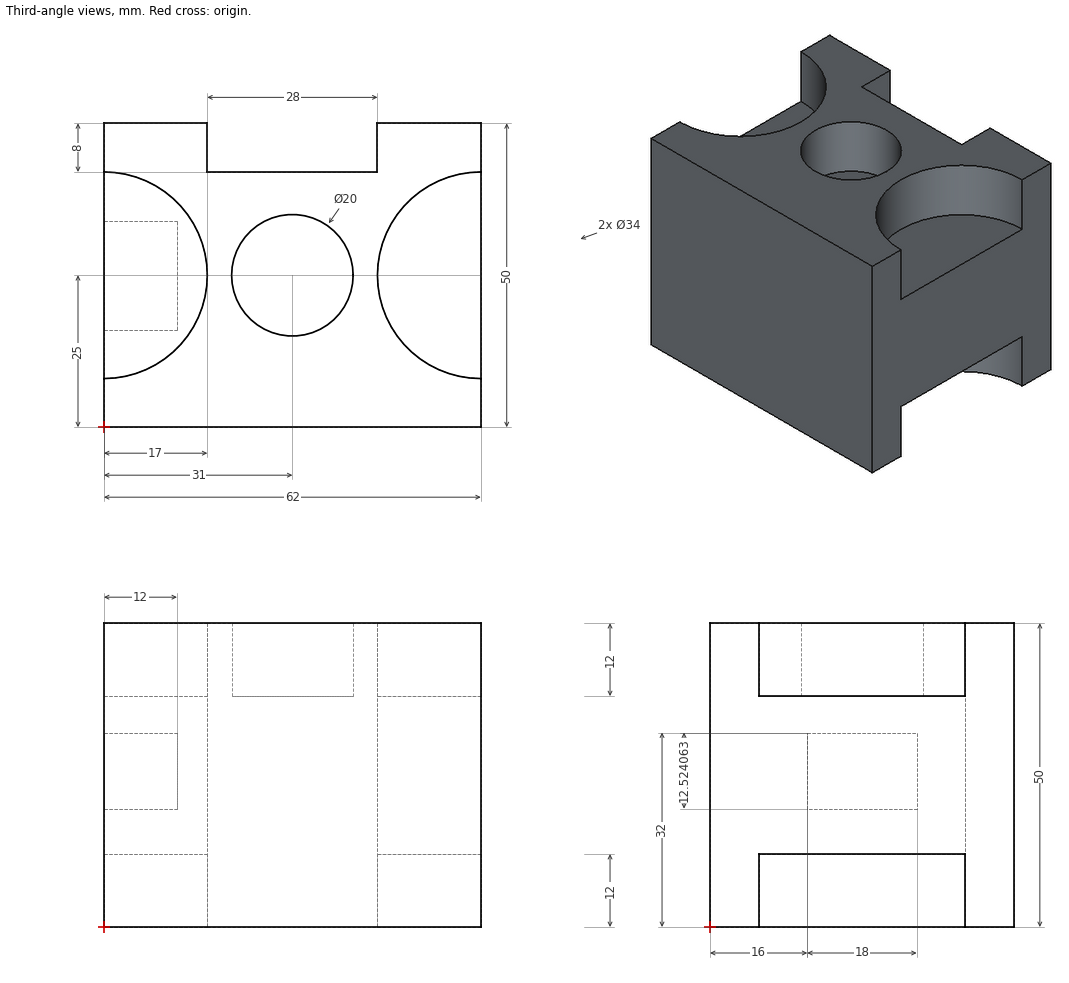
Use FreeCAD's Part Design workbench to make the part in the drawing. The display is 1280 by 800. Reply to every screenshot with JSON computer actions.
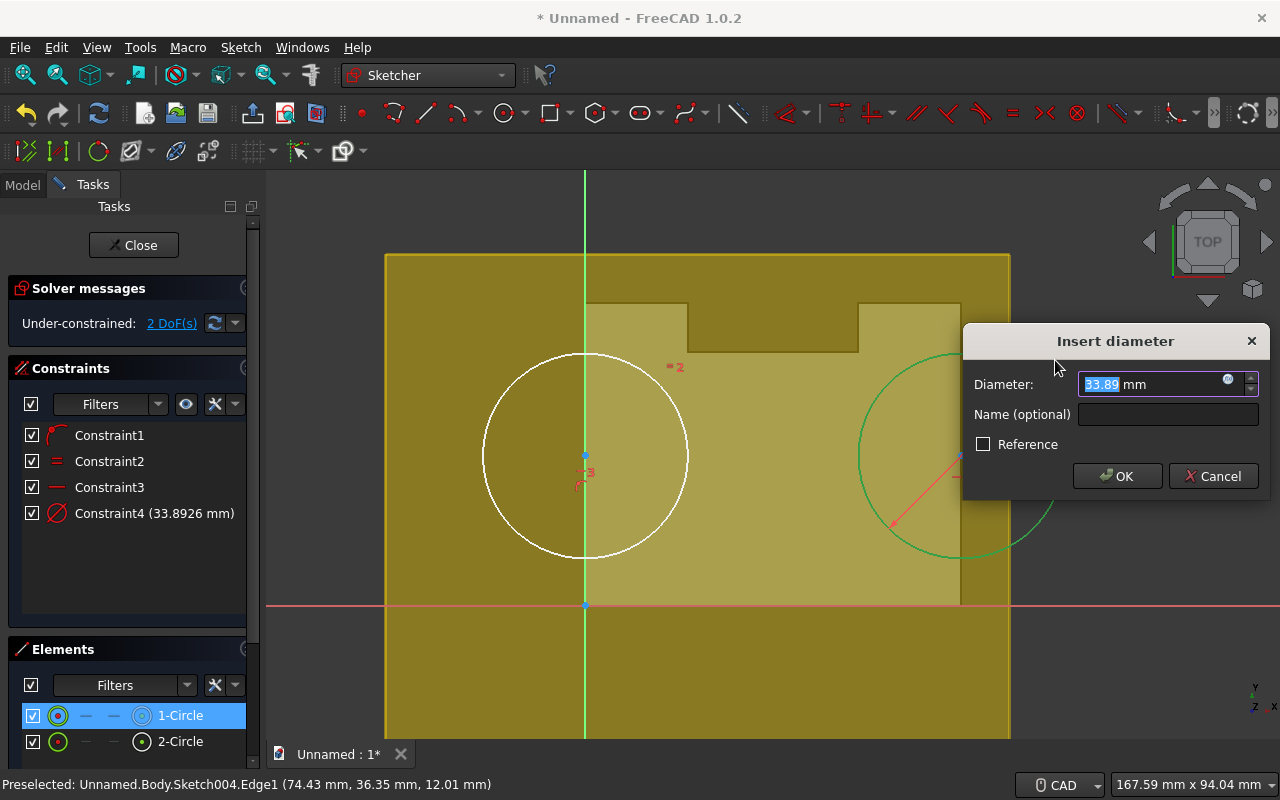
{"action": "type", "text": "34"}
{"action": "key", "text": "Return"}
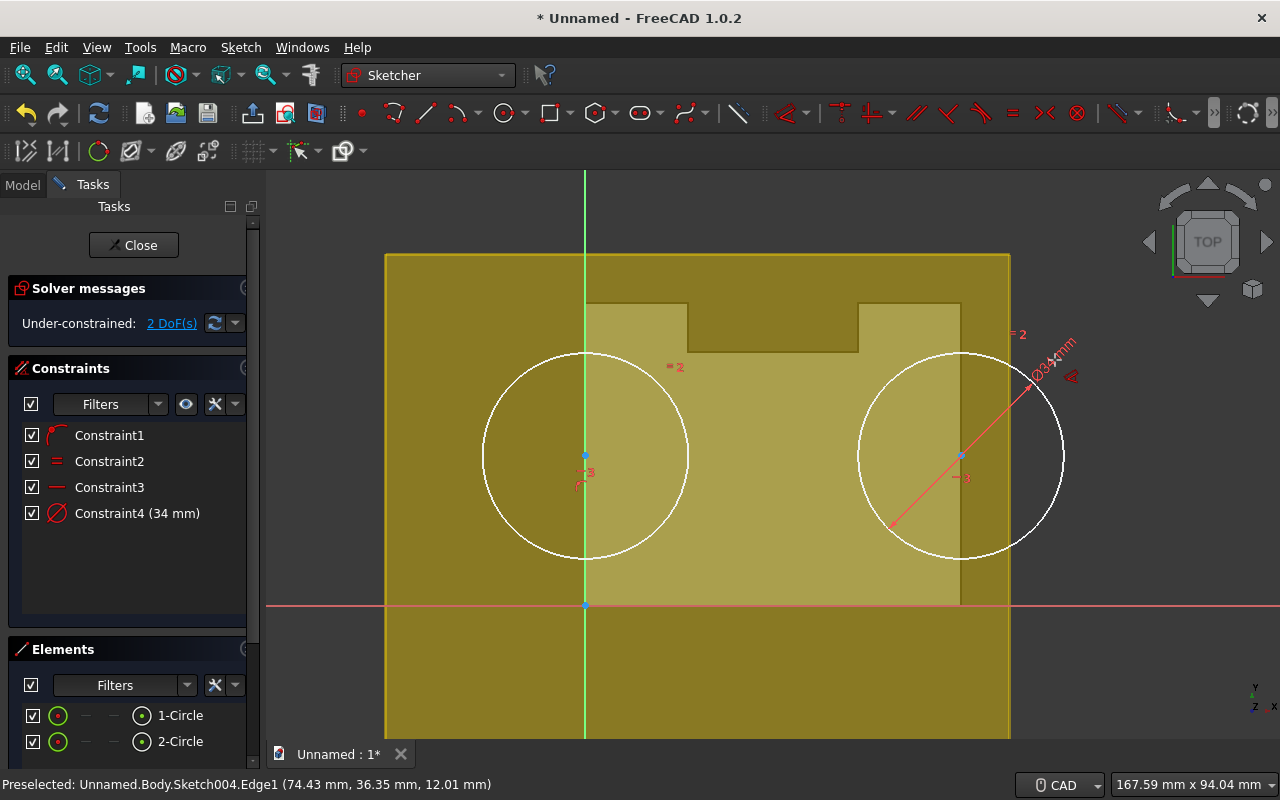
{"action": "left_click", "coordinate": [961, 456]}
{"action": "left_click", "coordinate": [773, 640]}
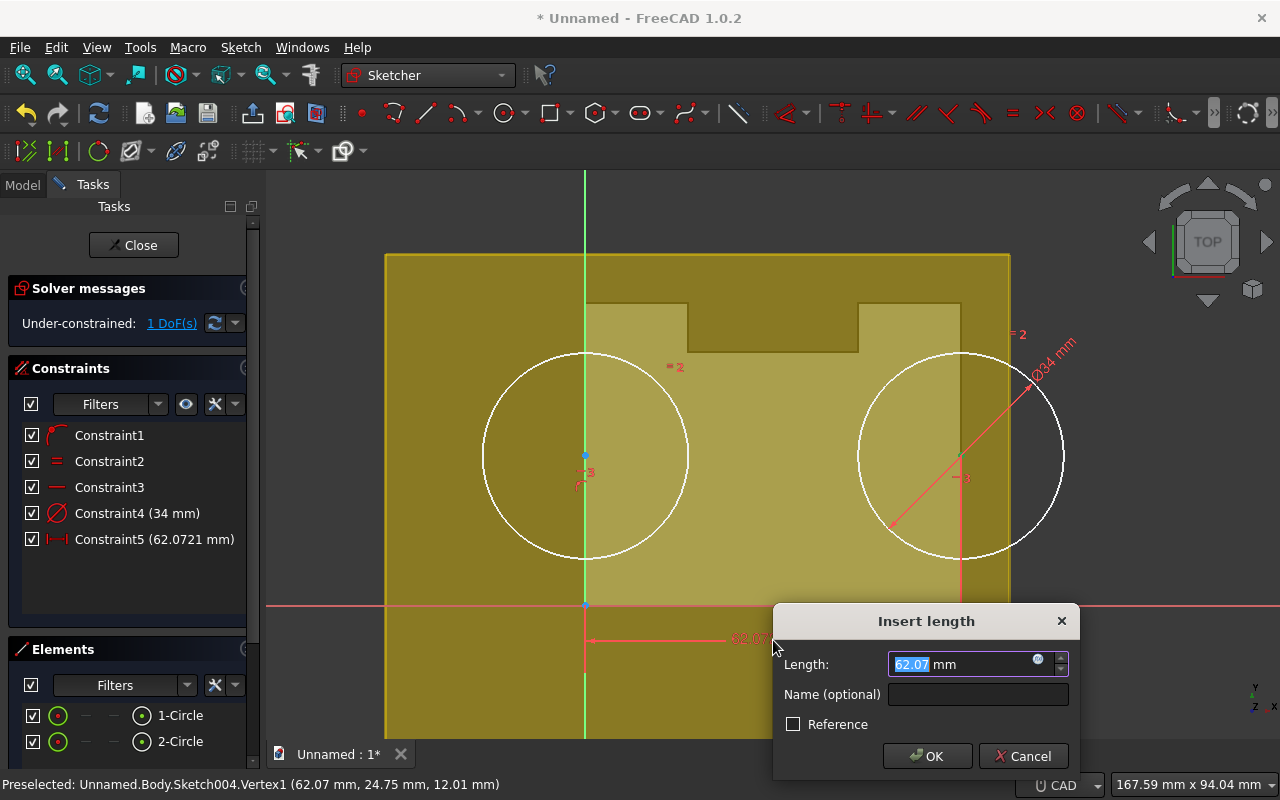
{"action": "type", "text": "62"}
{"action": "key", "text": "Return"}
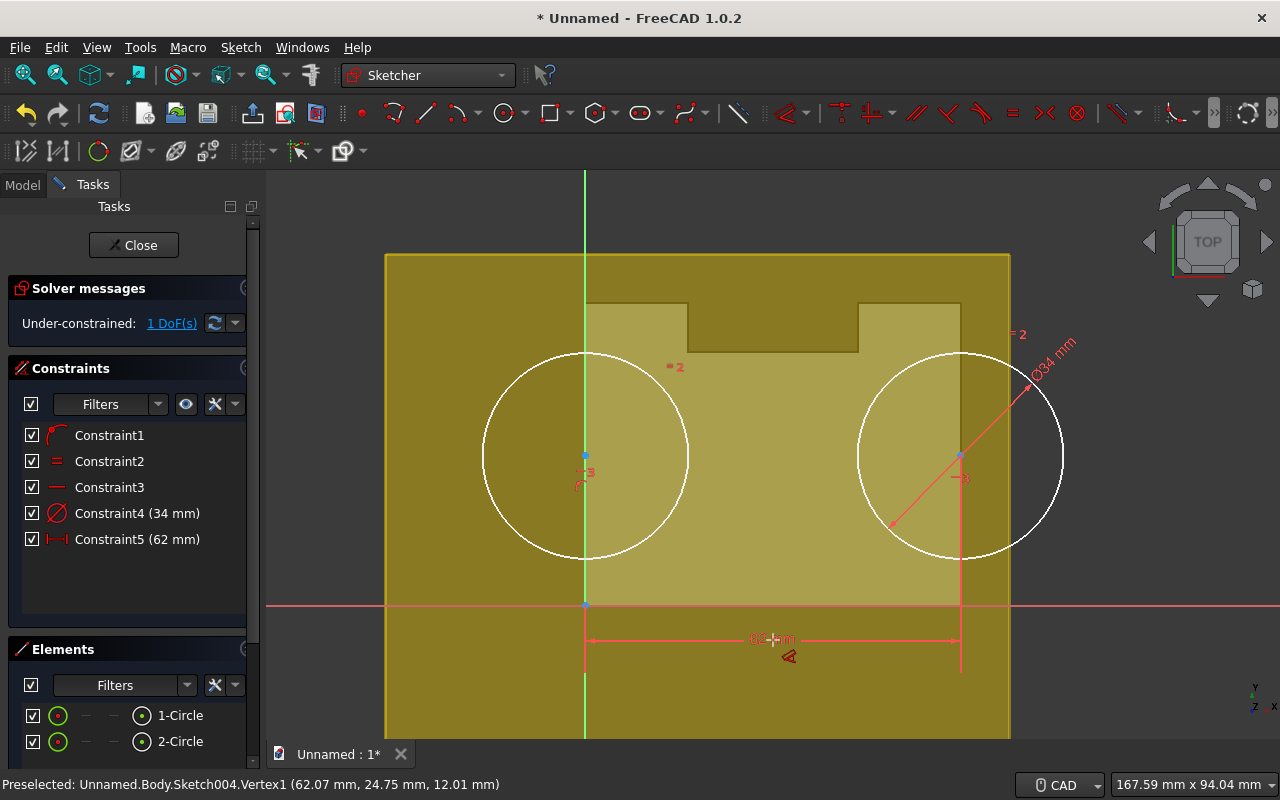
{"action": "left_click", "coordinate": [961, 456]}
{"action": "left_click", "coordinate": [995, 531]}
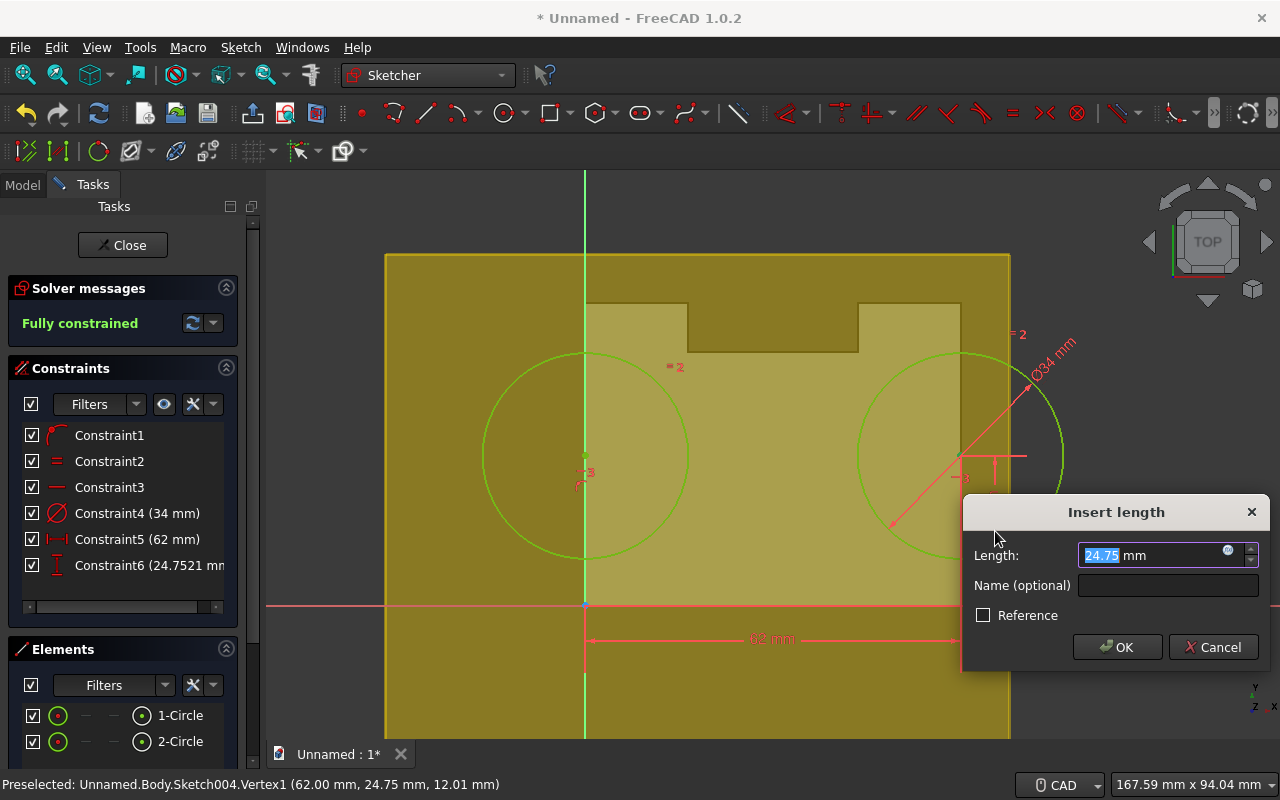
{"action": "type", "text": "25"}
{"action": "key", "text": "Return"}
{"action": "key", "text": "Escape"}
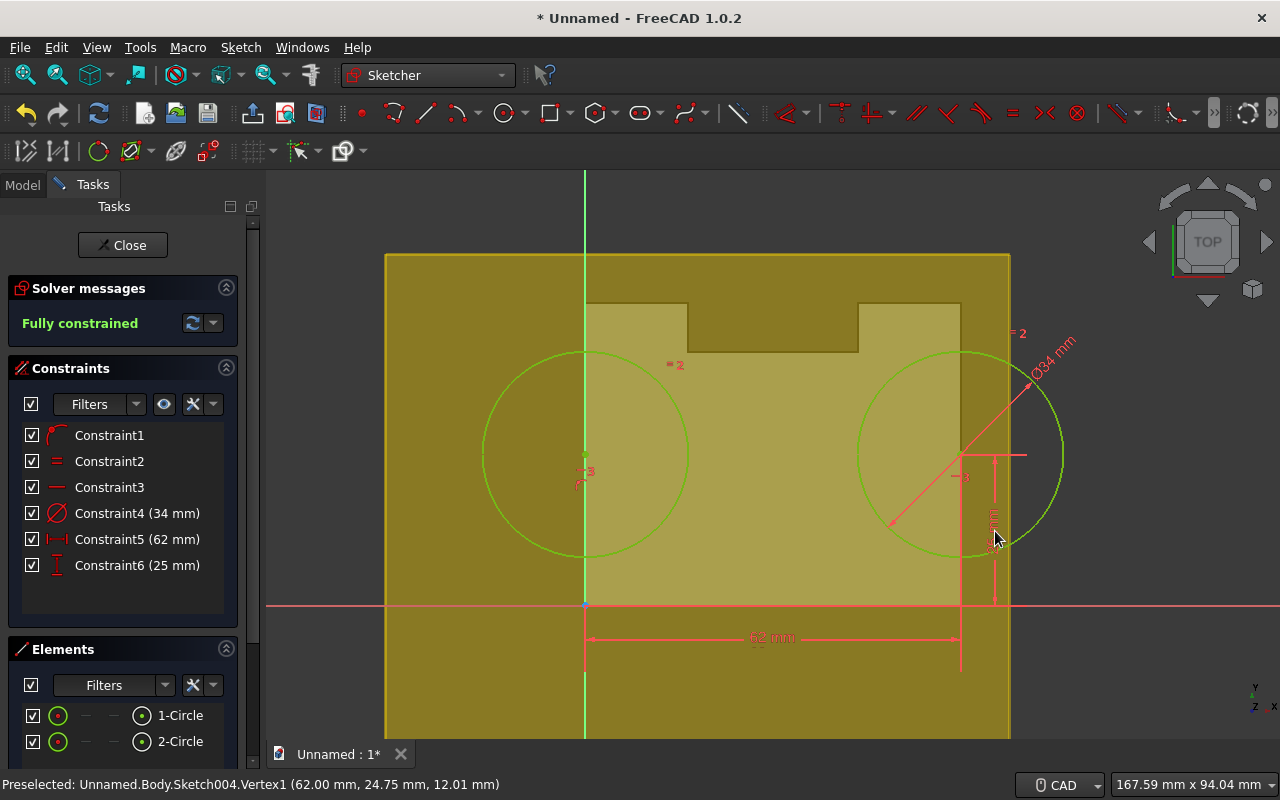
{"action": "left_click", "coordinate": [123, 245]}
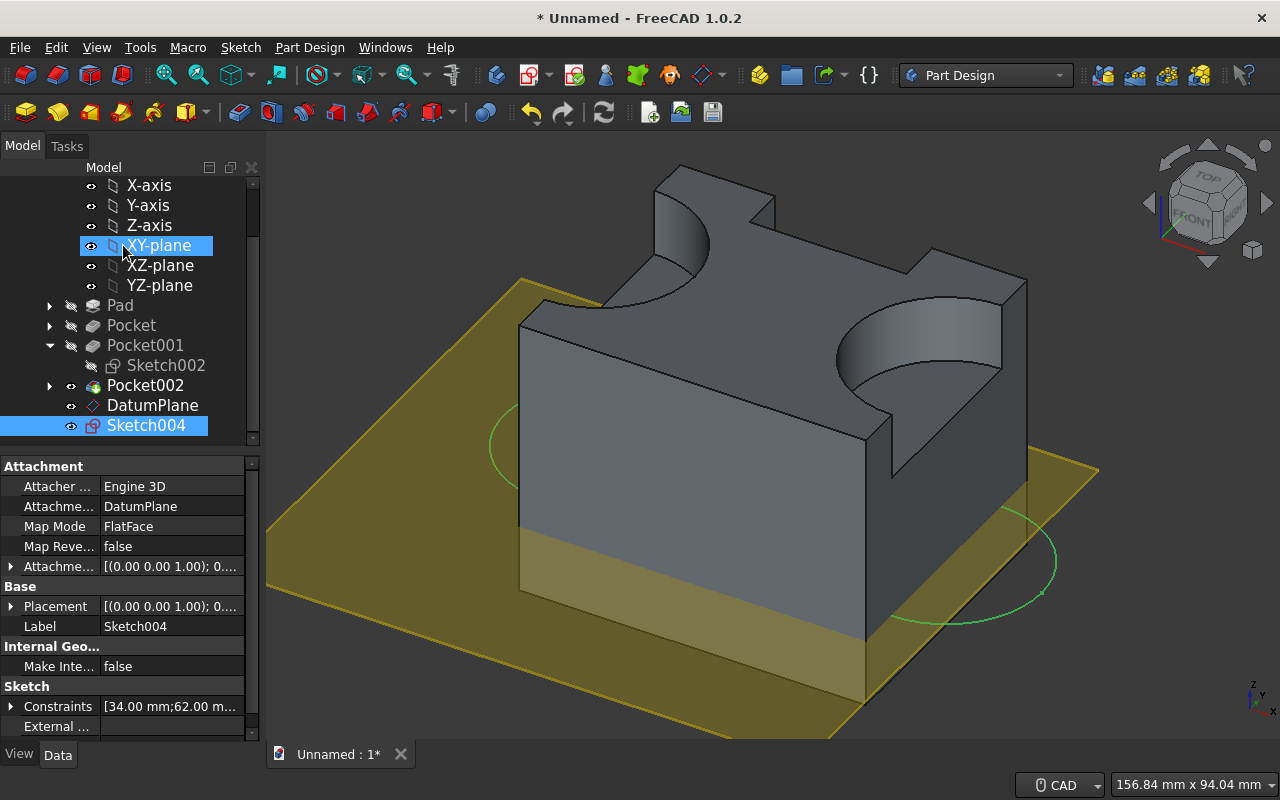
{"action": "left_click", "coordinate": [240, 112]}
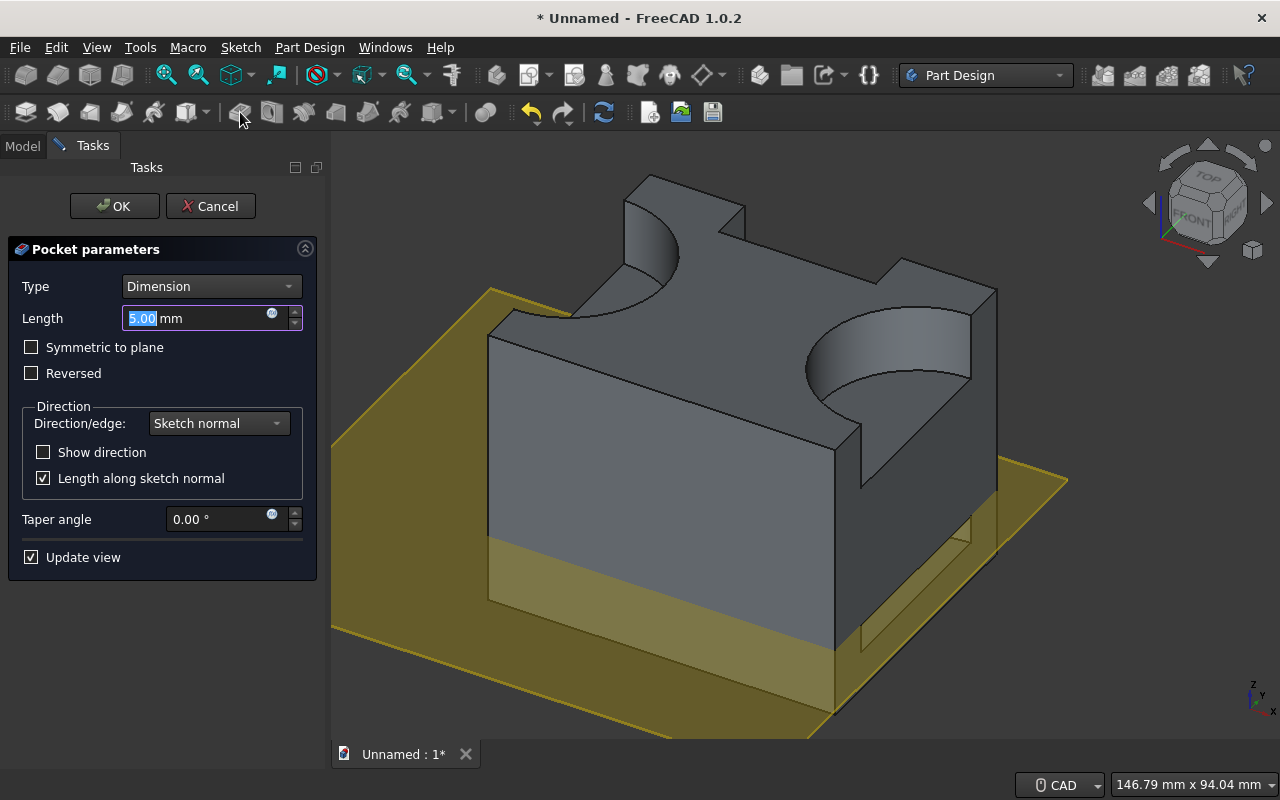
{"action": "type", "text": "12"}
{"action": "key", "text": "Tab"}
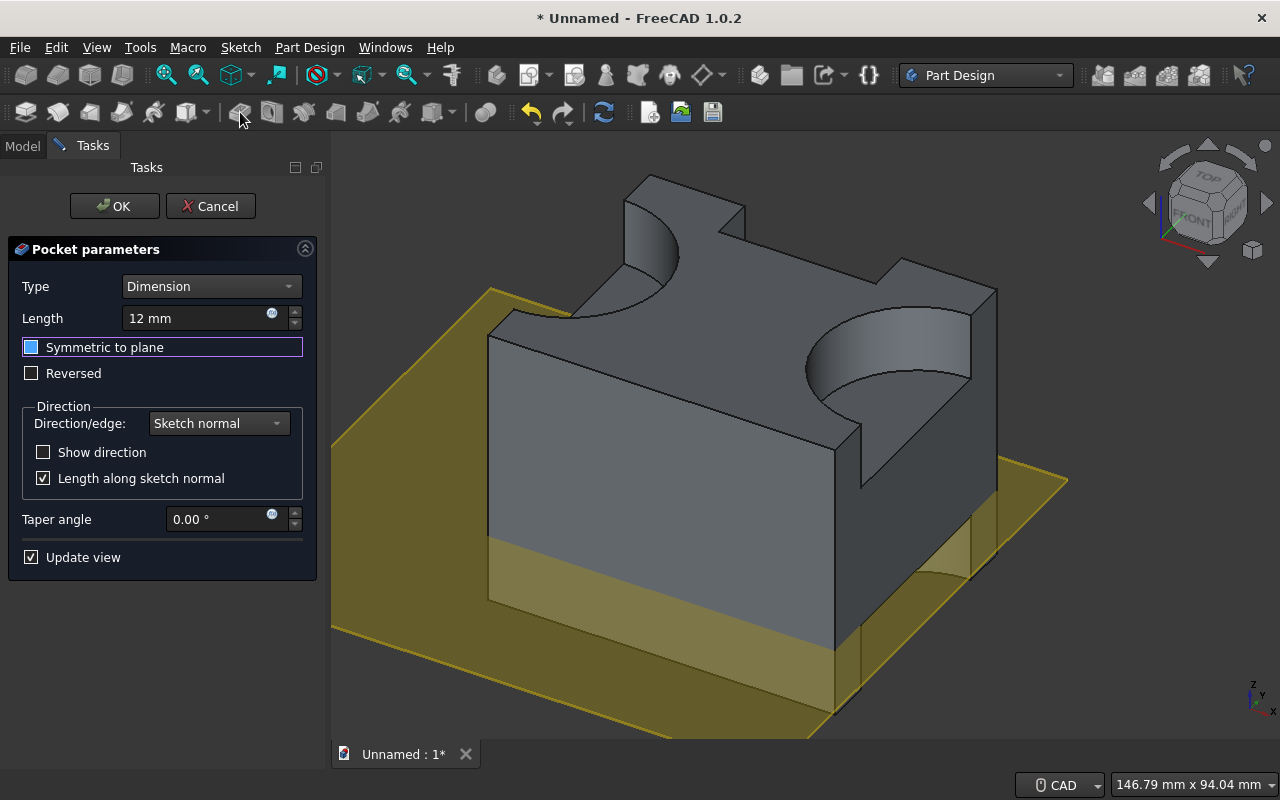
{"action": "left_click", "coordinate": [115, 206]}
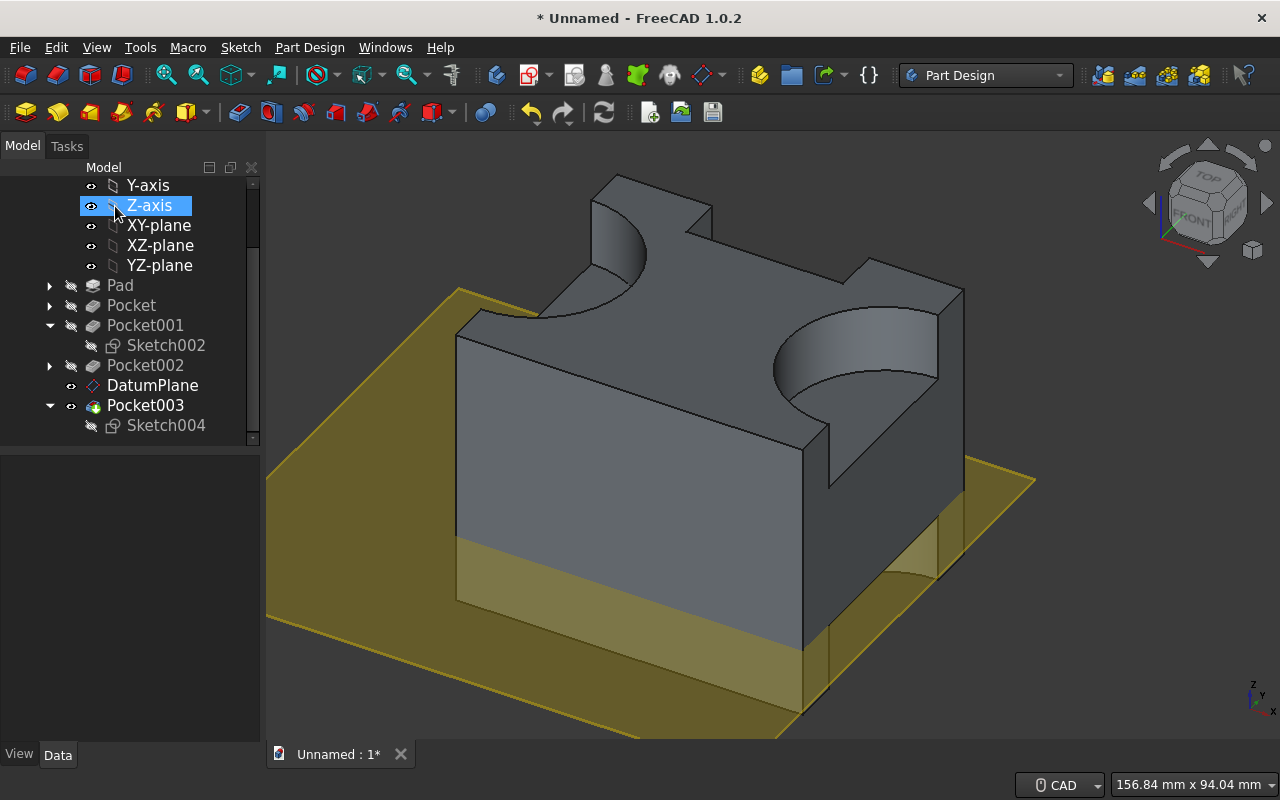
{"action": "left_click", "coordinate": [116, 386]}
{"action": "key", "text": "space"}